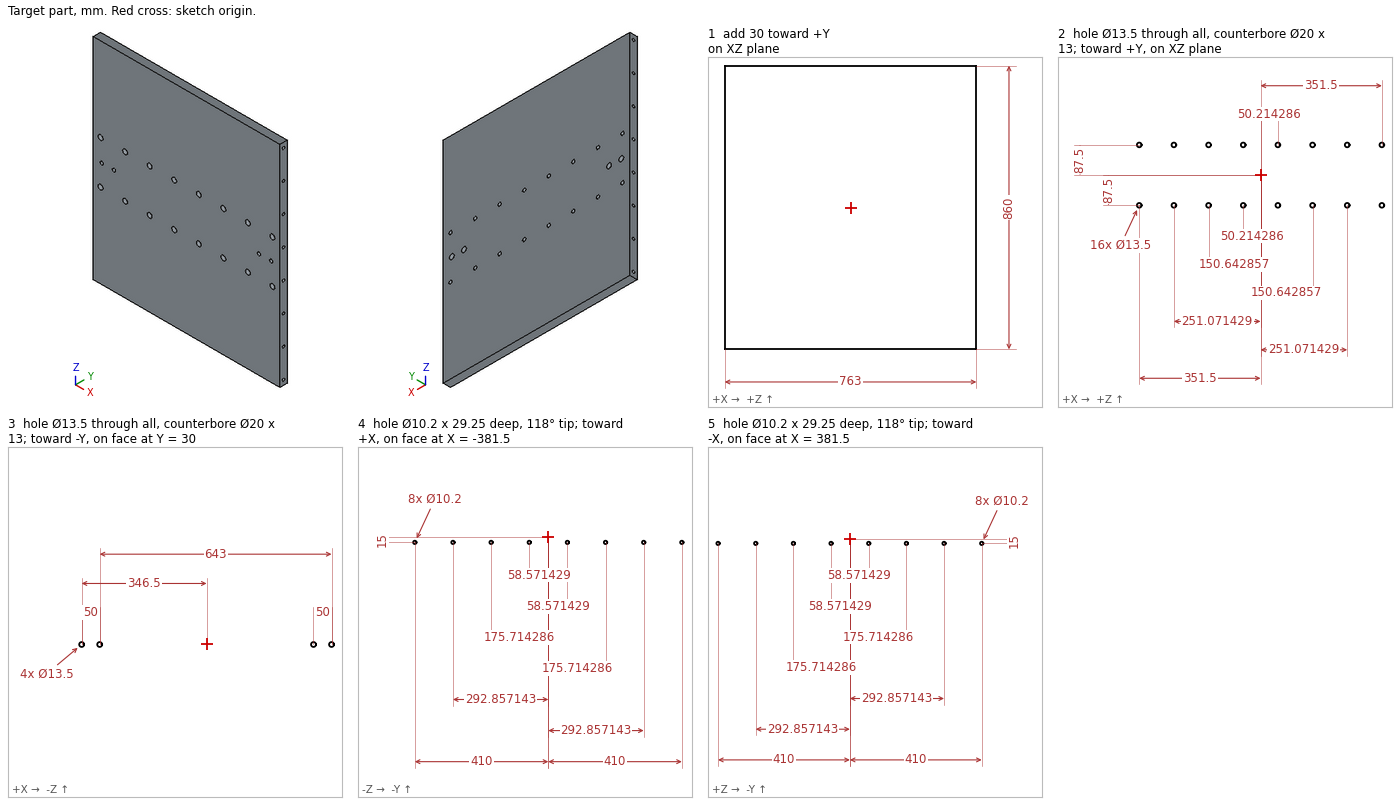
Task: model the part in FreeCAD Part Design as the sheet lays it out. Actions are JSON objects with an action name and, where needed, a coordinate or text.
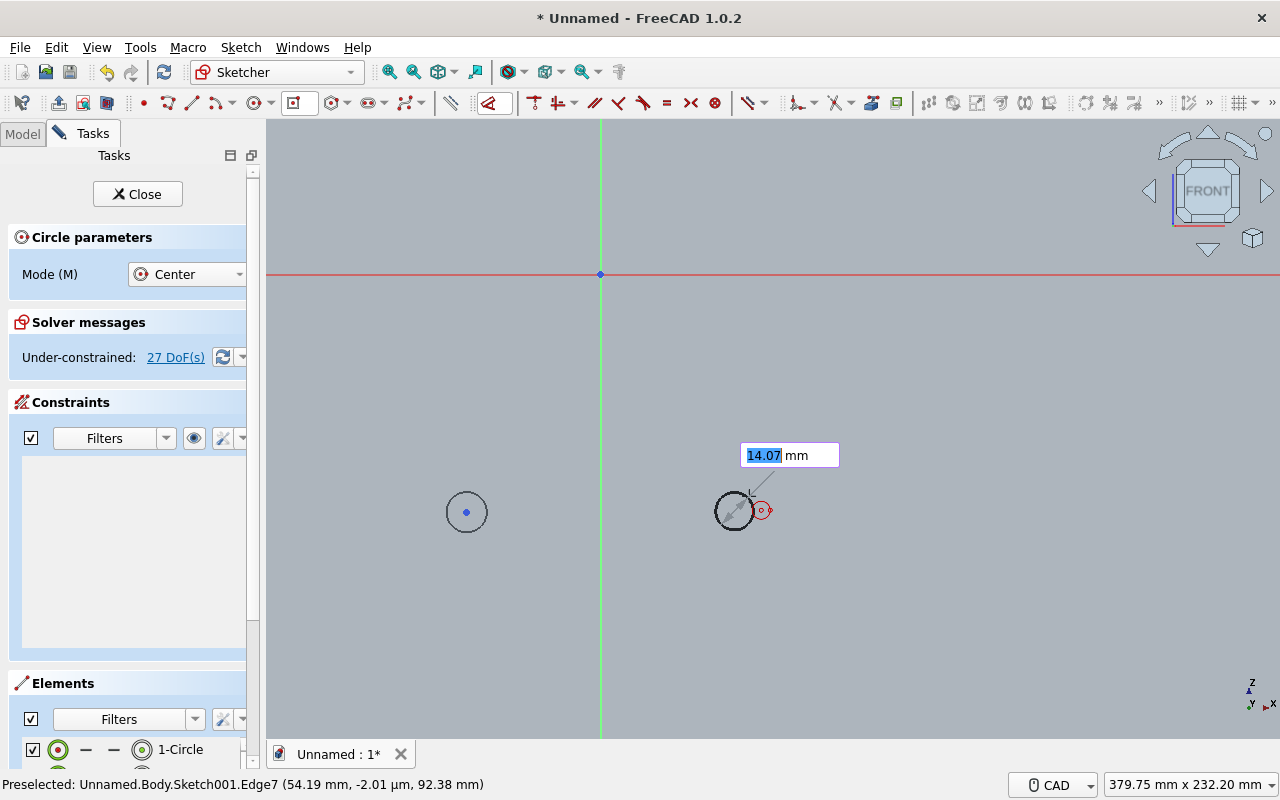
{"action": "left_click", "coordinate": [748, 496]}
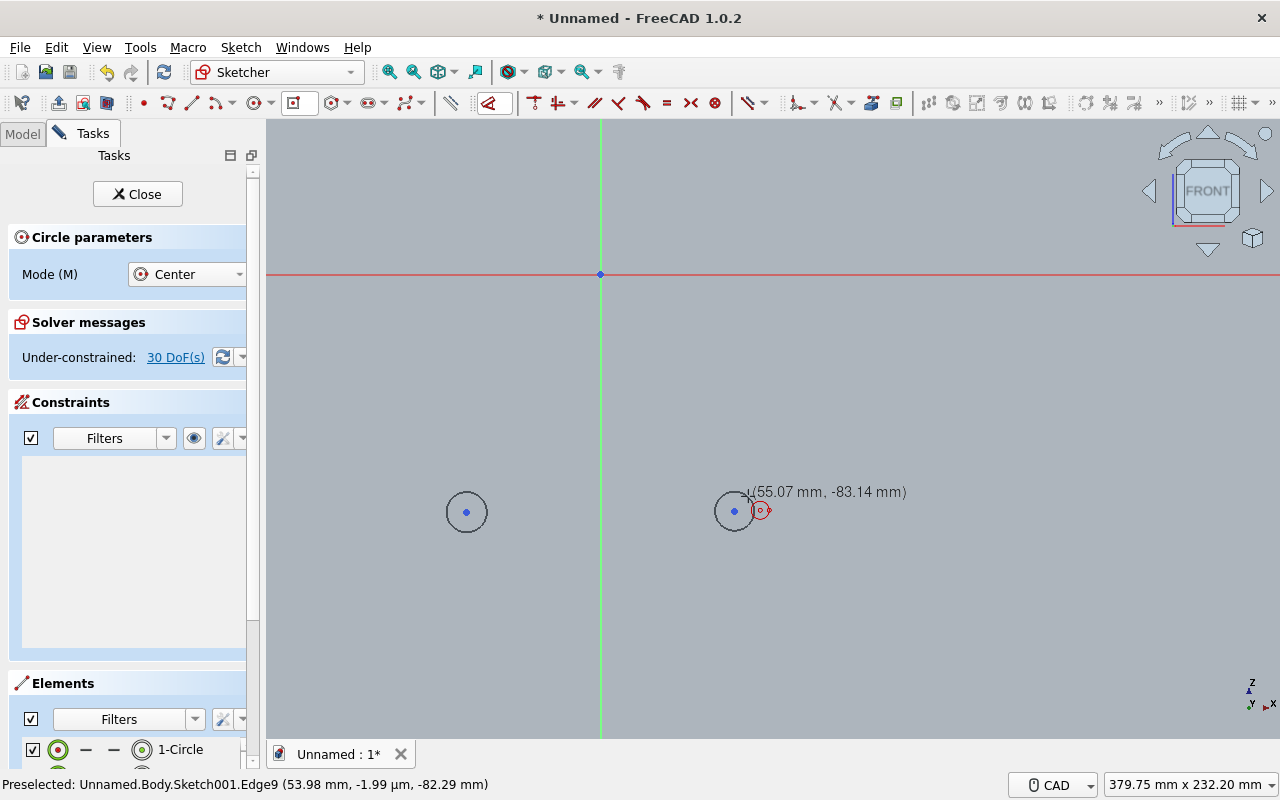
{"action": "scroll", "coordinate": [1003, 509], "scroll_direction": "up", "scroll_amount": 2}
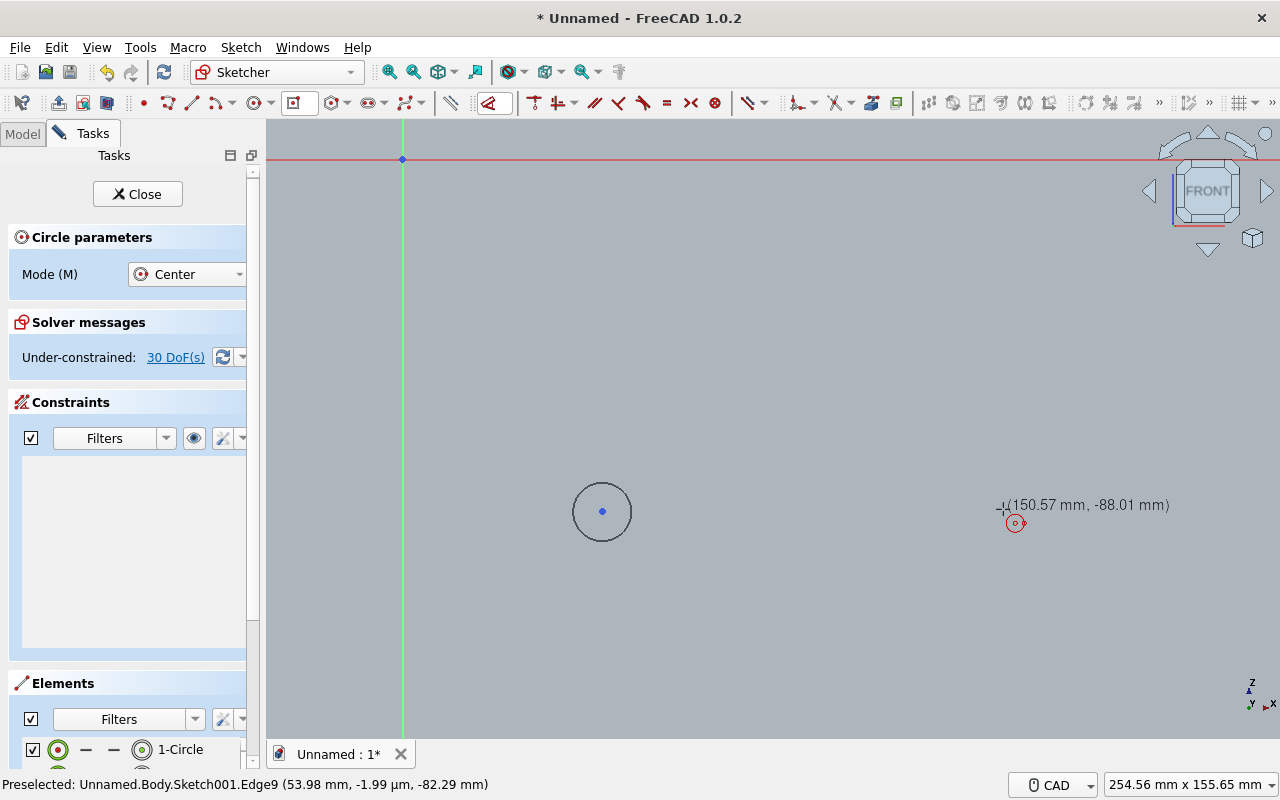
{"action": "scroll", "coordinate": [781, 497], "scroll_direction": "down", "scroll_amount": 8}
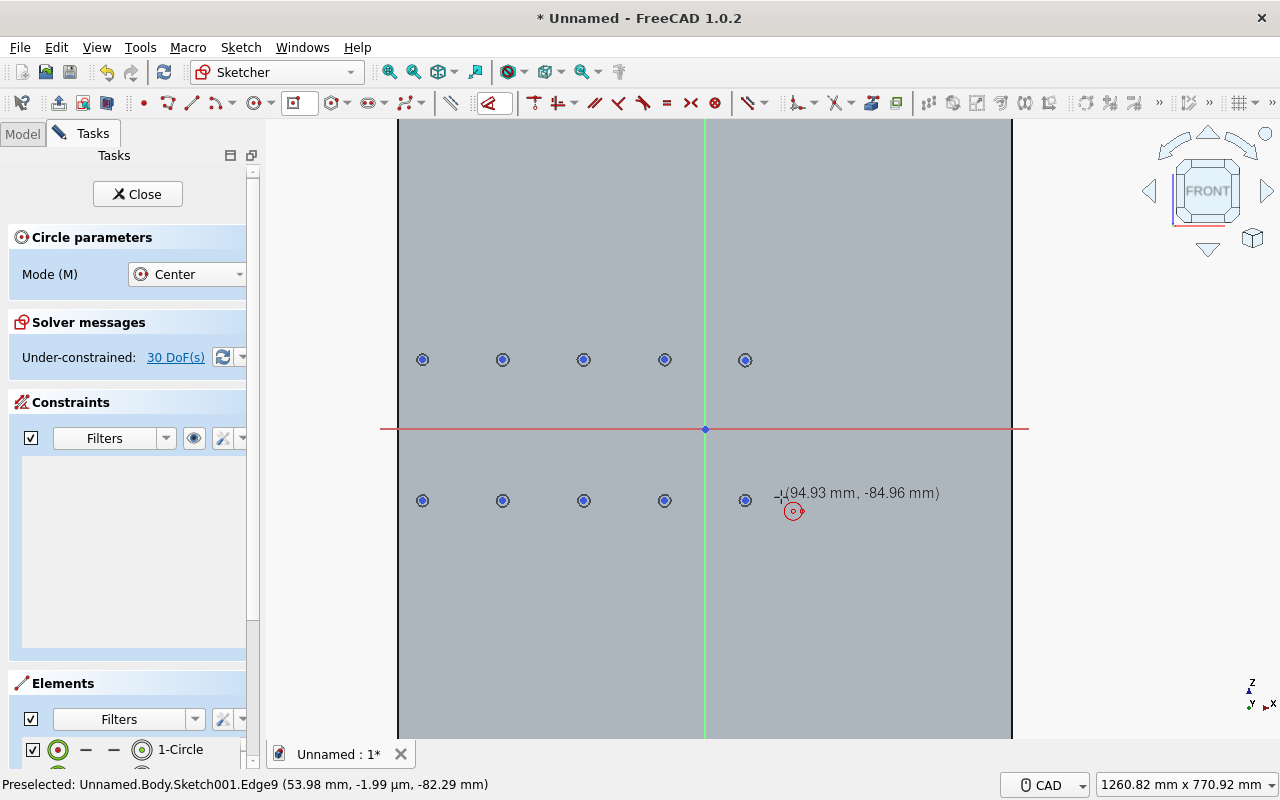
{"action": "left_click", "coordinate": [826, 500]}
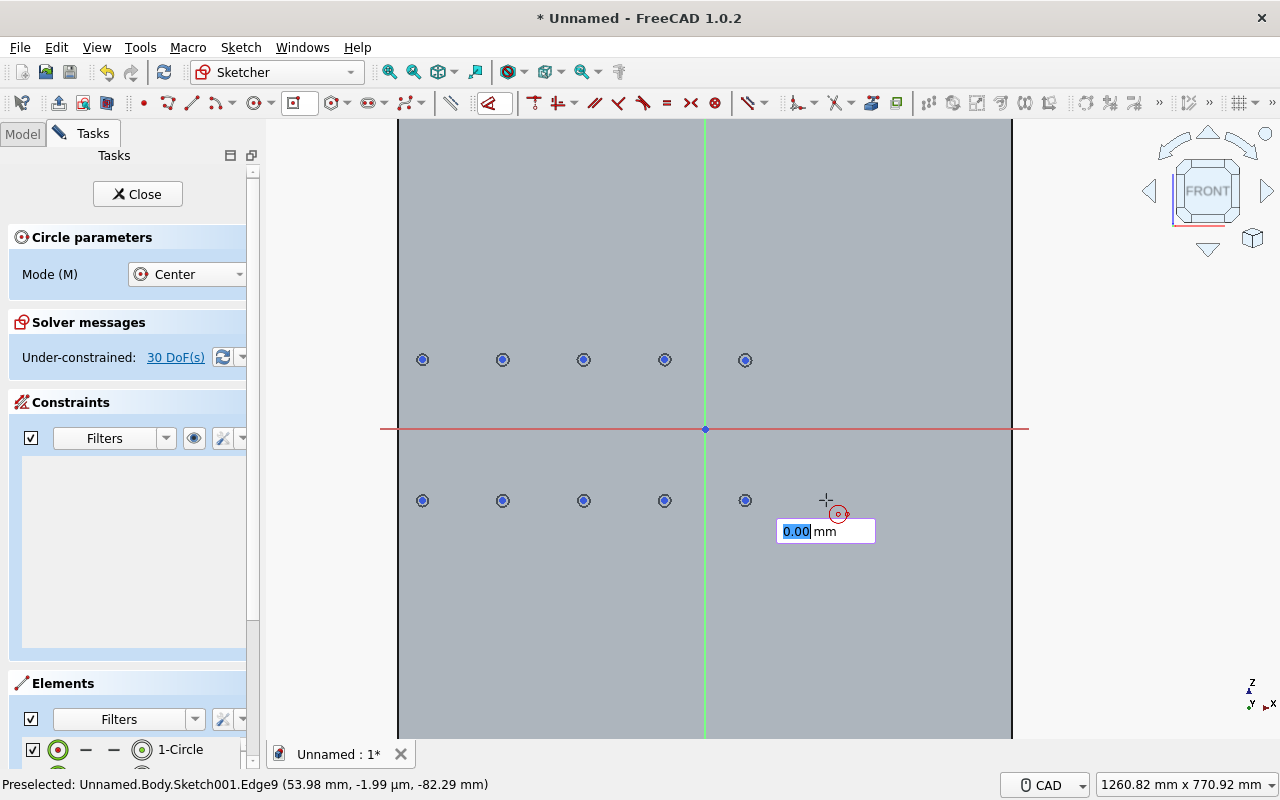
{"action": "scroll", "coordinate": [830, 496], "scroll_direction": "up", "scroll_amount": 6}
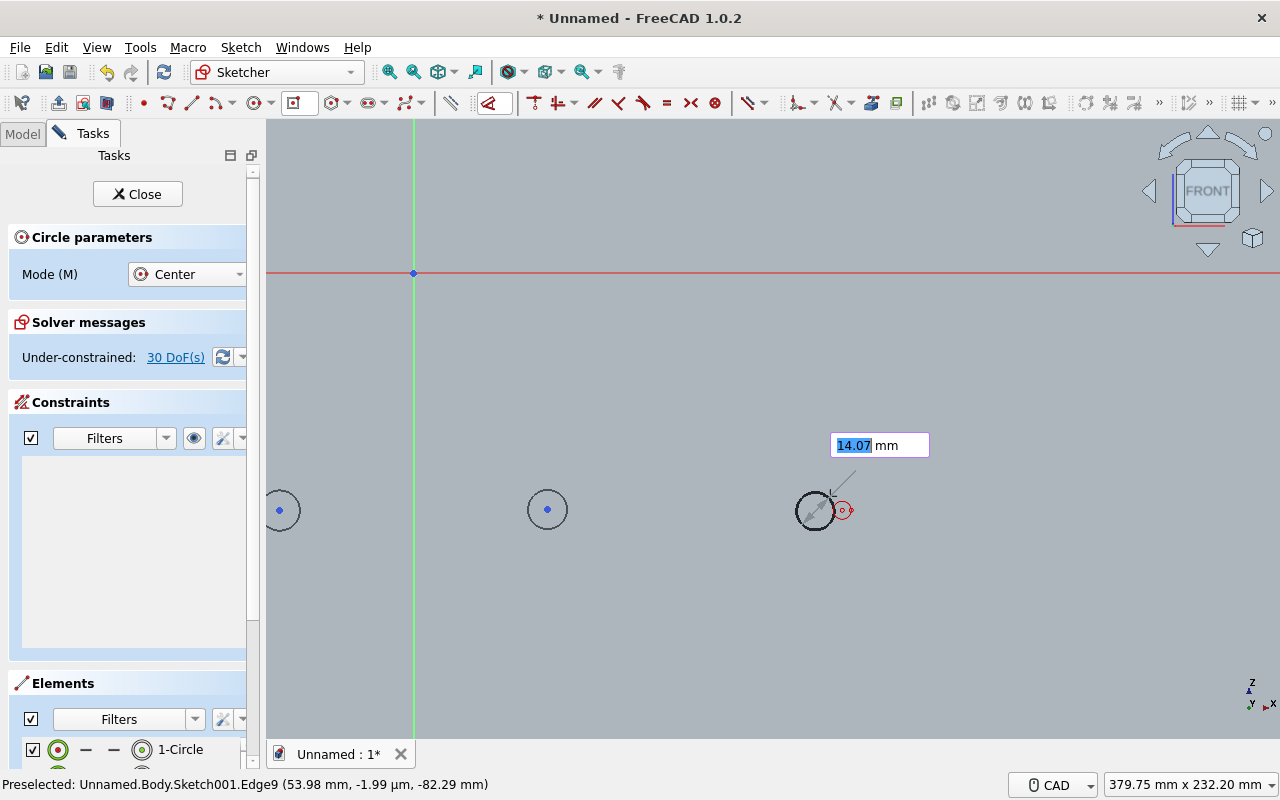
{"action": "left_click", "coordinate": [829, 494]}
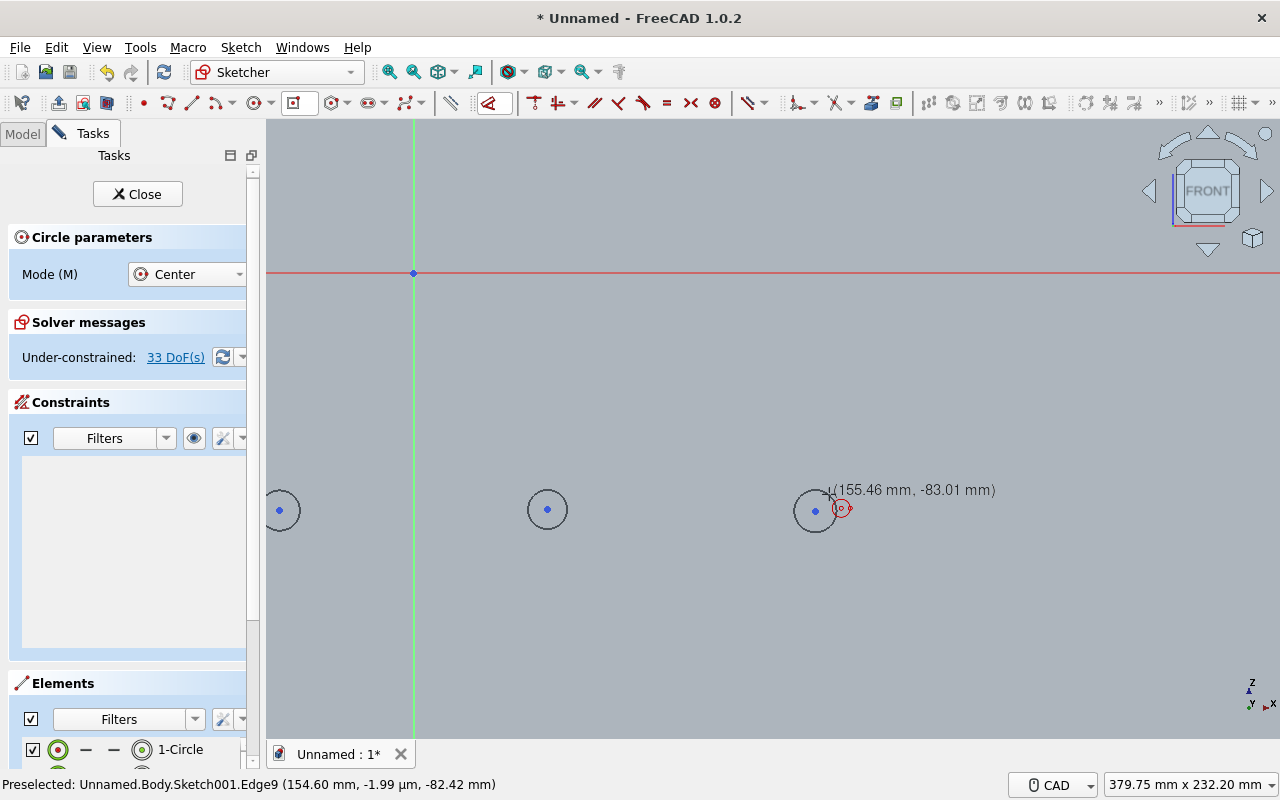
{"action": "scroll", "coordinate": [830, 496], "scroll_direction": "down", "scroll_amount": 6}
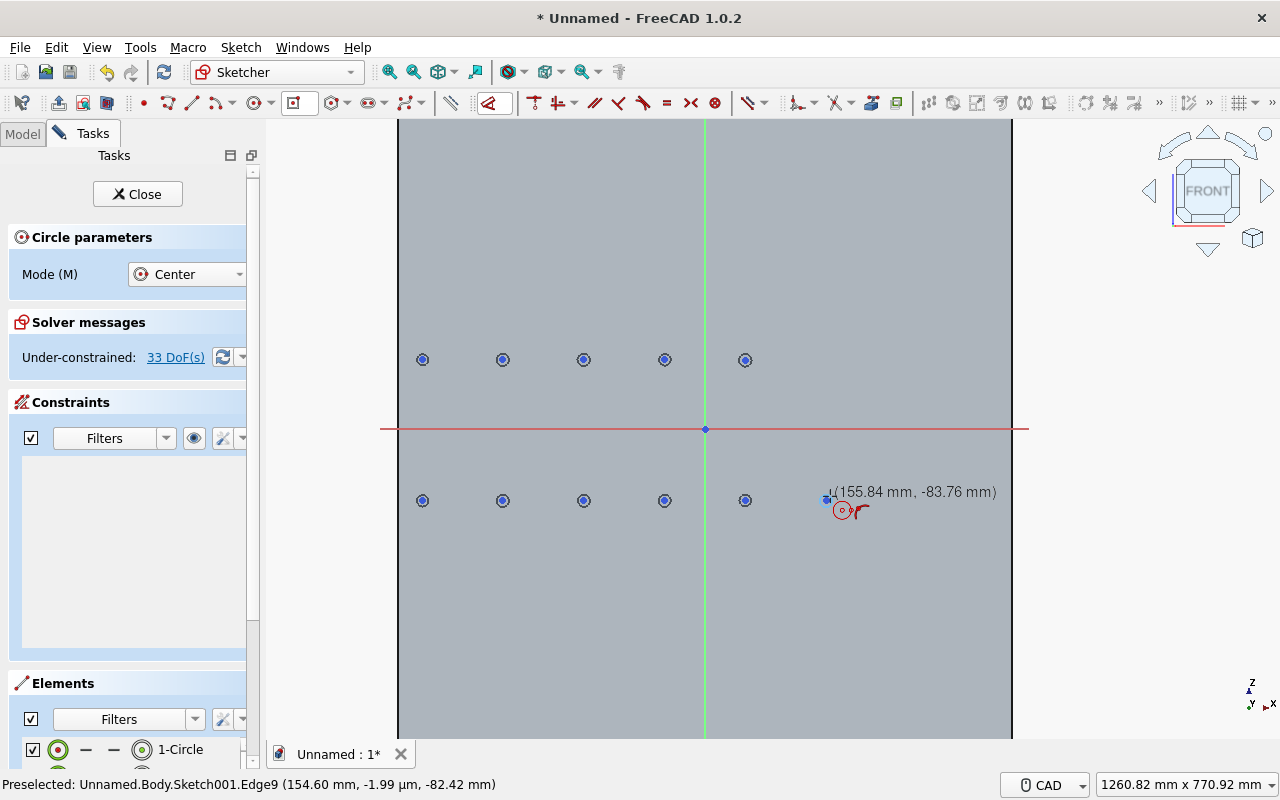
{"action": "scroll", "coordinate": [826, 359], "scroll_direction": "up", "scroll_amount": 8}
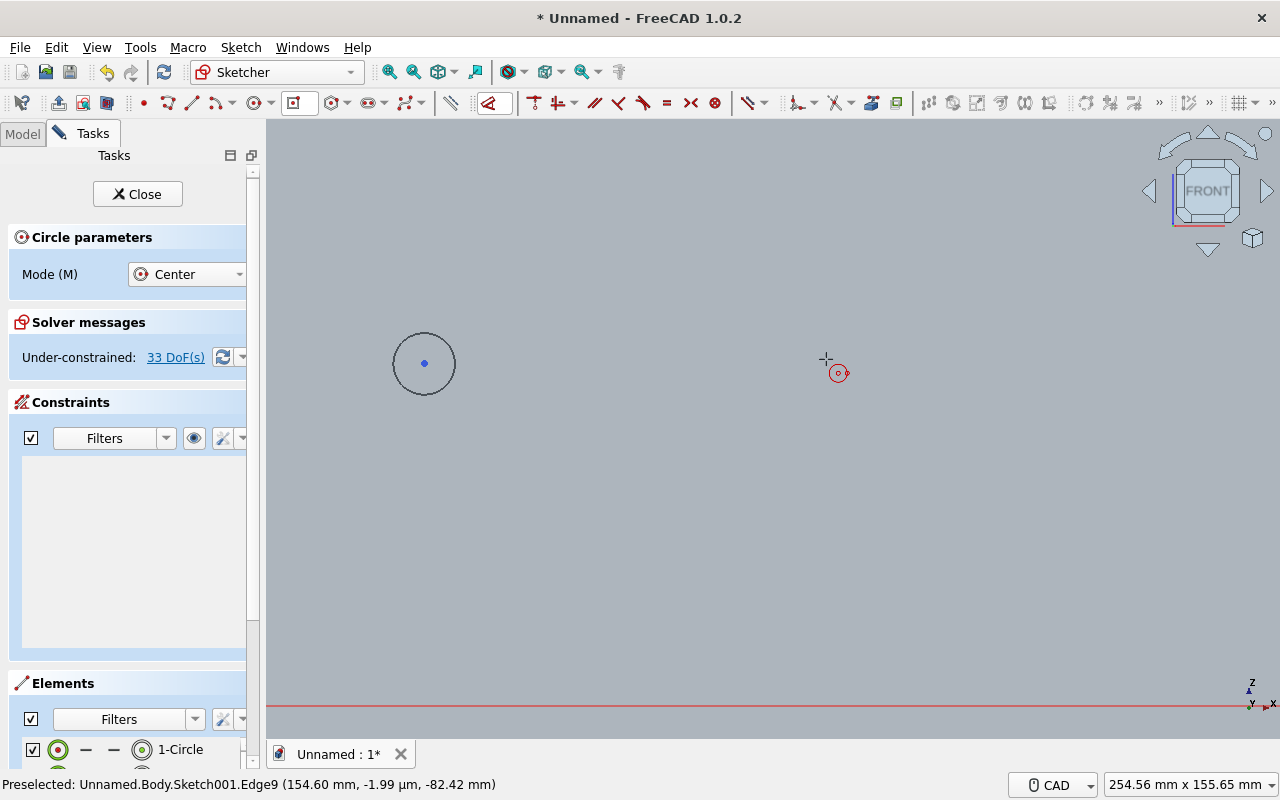
{"action": "scroll", "coordinate": [826, 359], "scroll_direction": "down", "scroll_amount": 8}